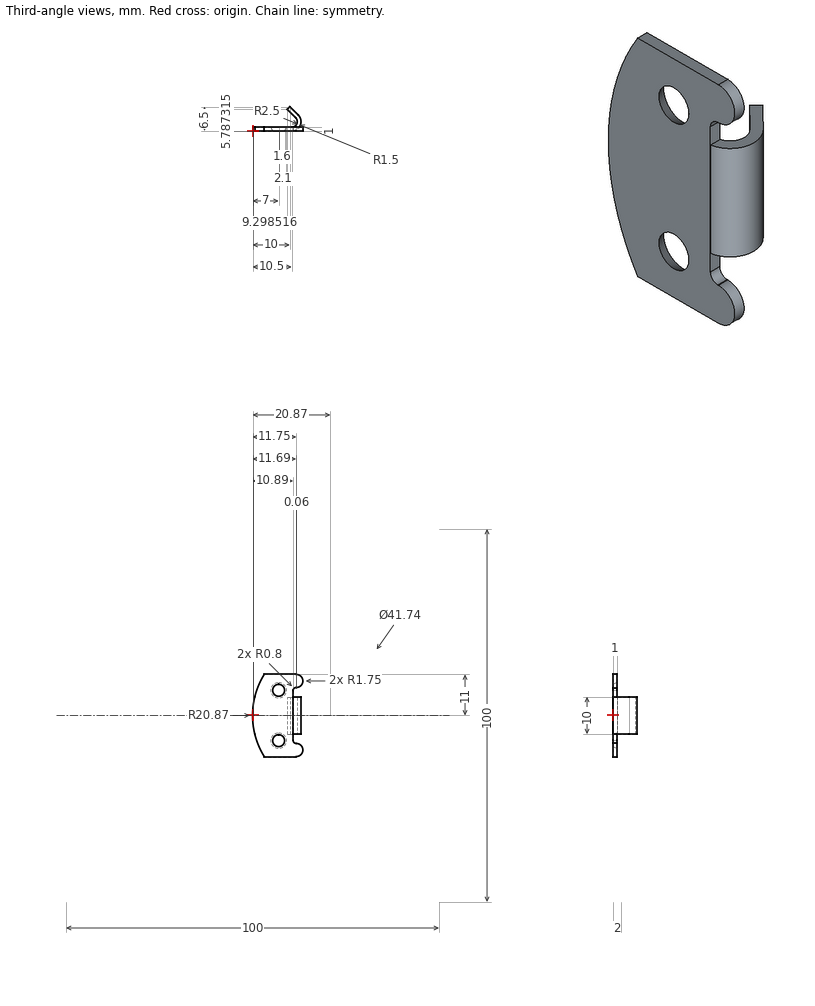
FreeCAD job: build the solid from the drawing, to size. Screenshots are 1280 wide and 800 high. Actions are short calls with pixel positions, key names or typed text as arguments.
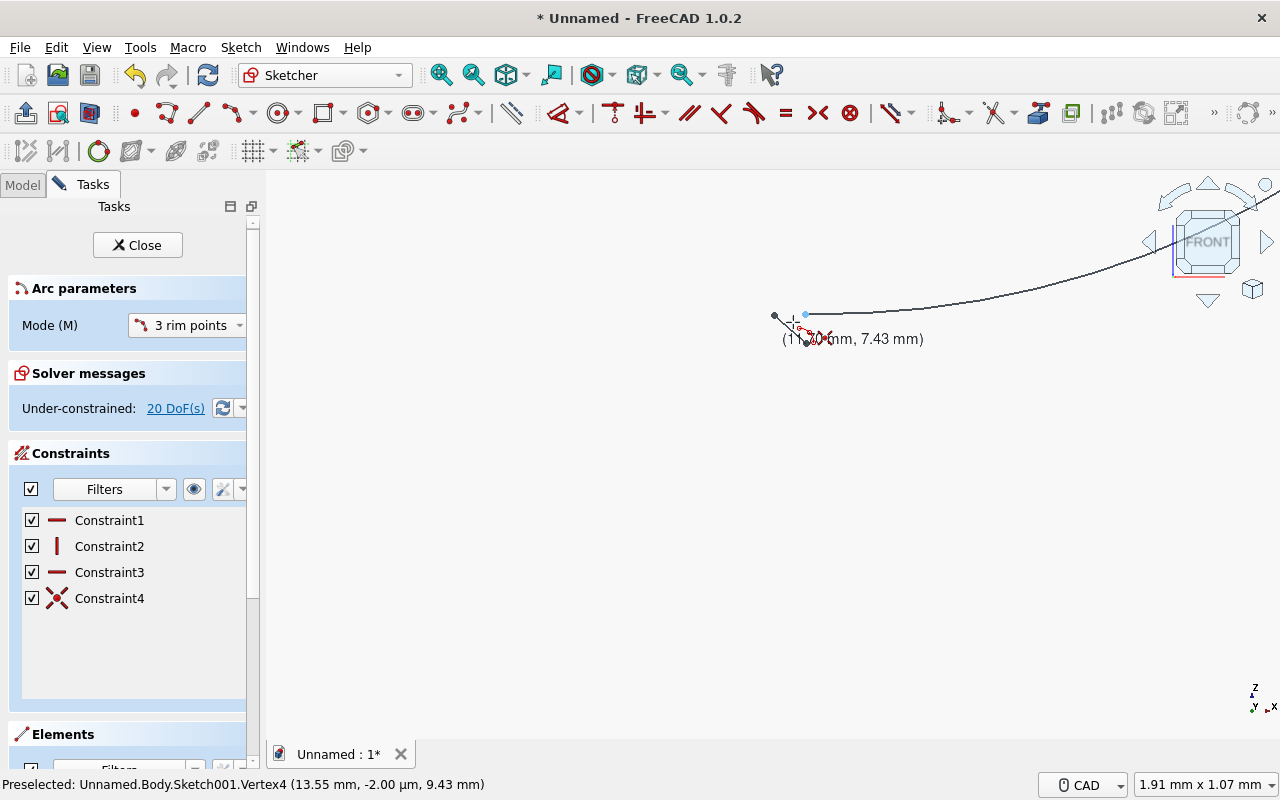
click(774, 315)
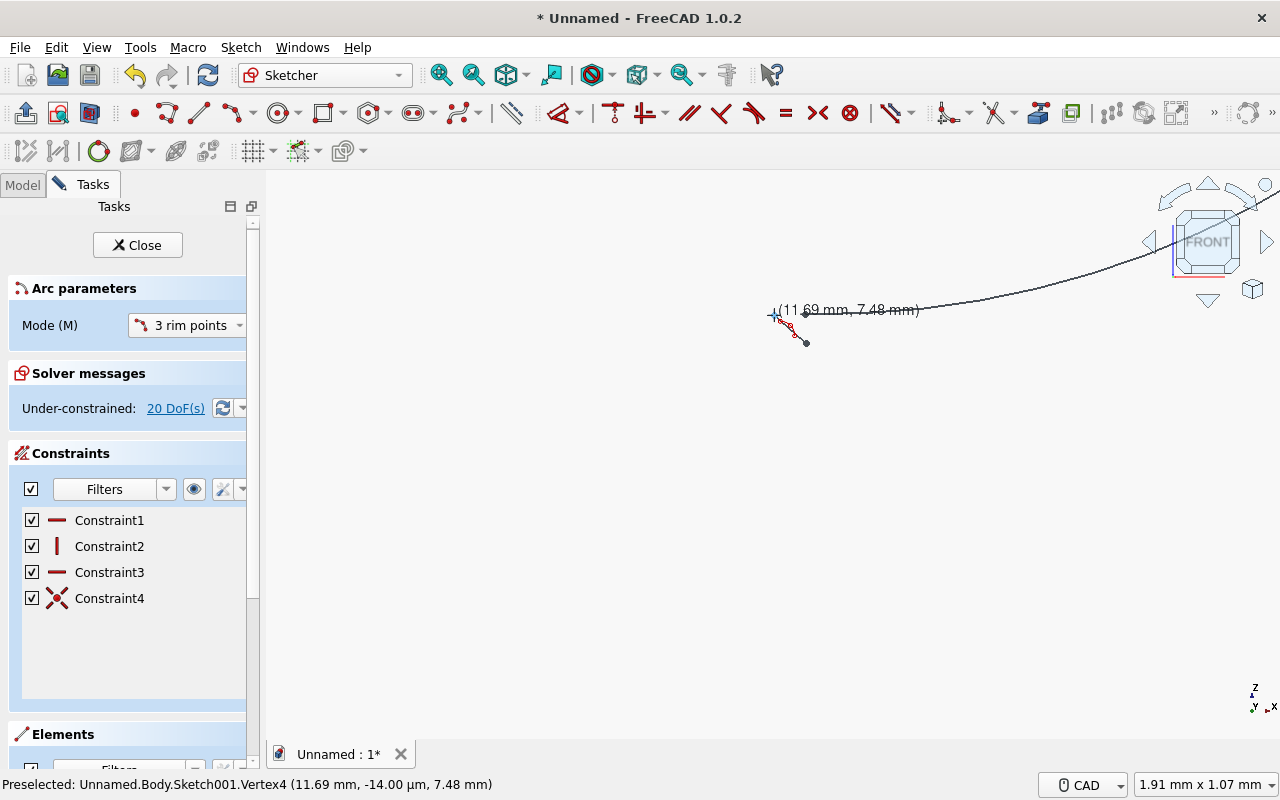
scroll(793, 322, down, 17)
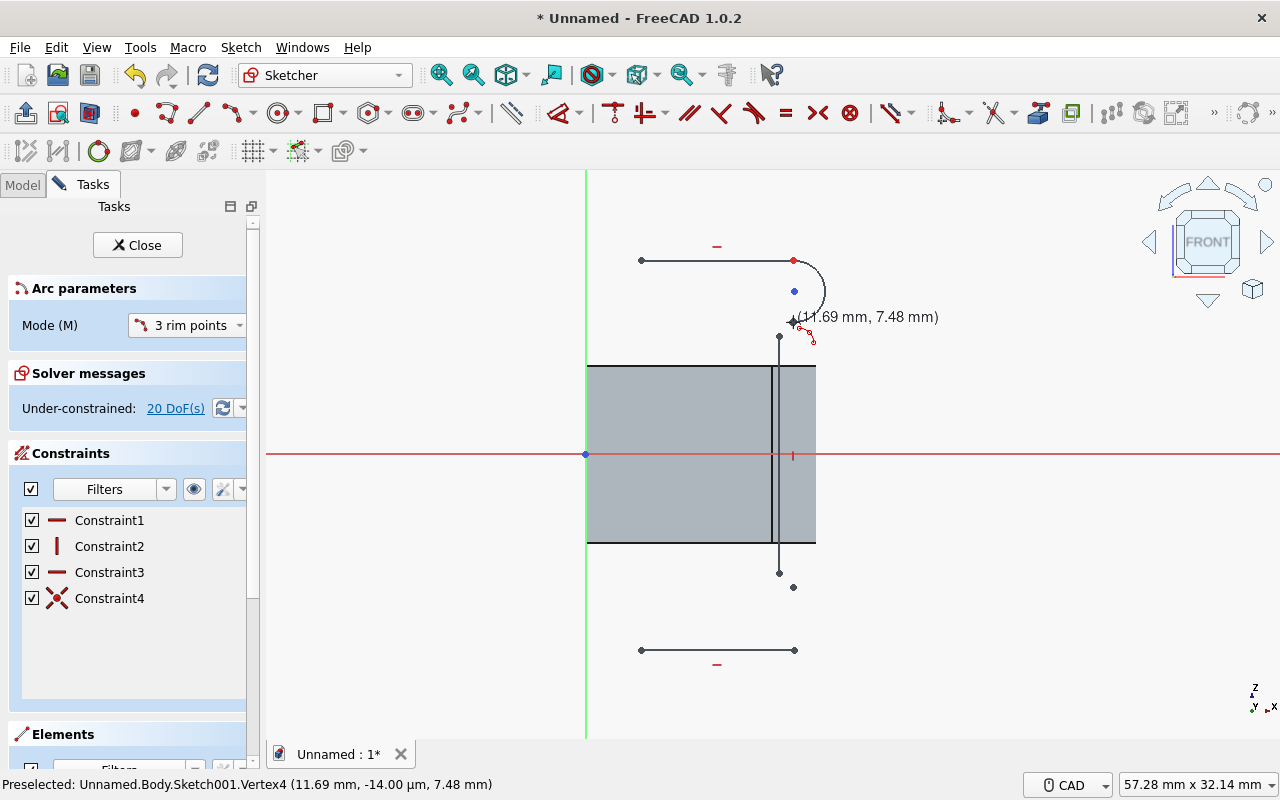
click(779, 337)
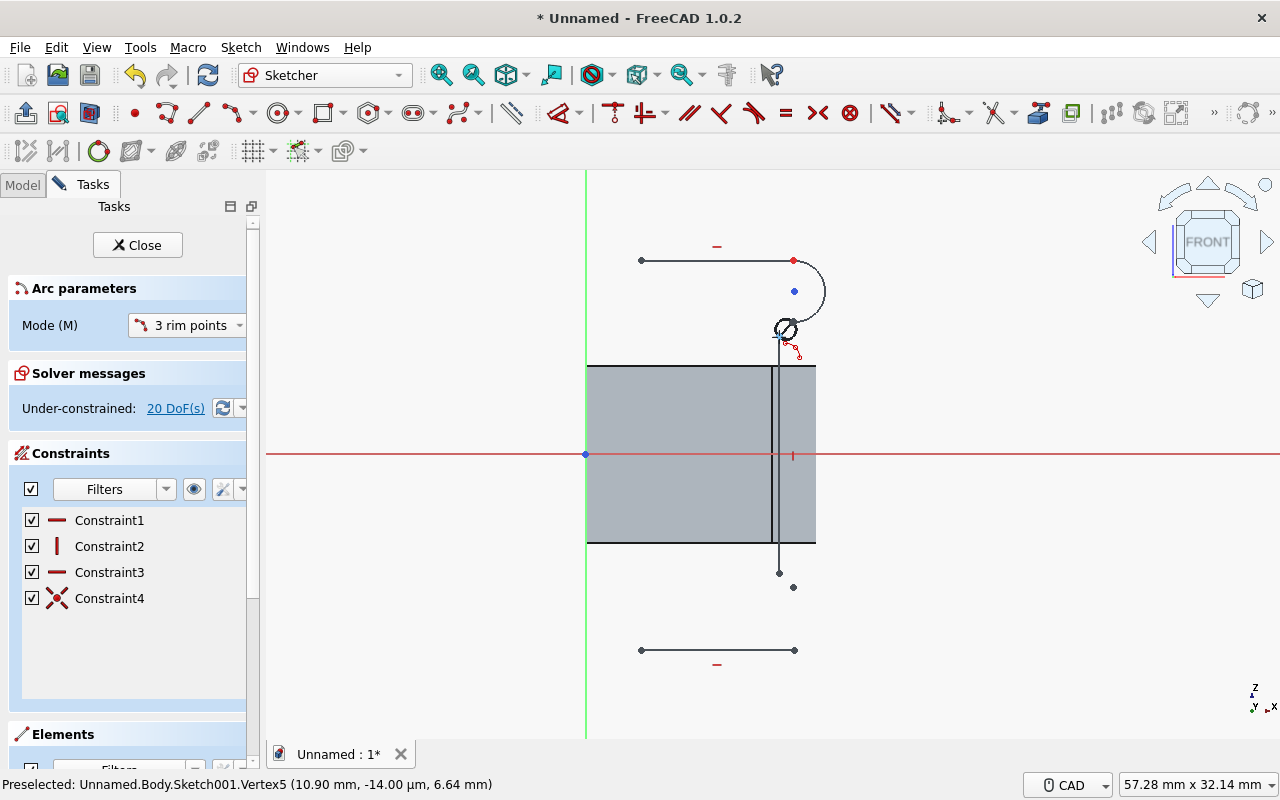
scroll(783, 326, up, 7)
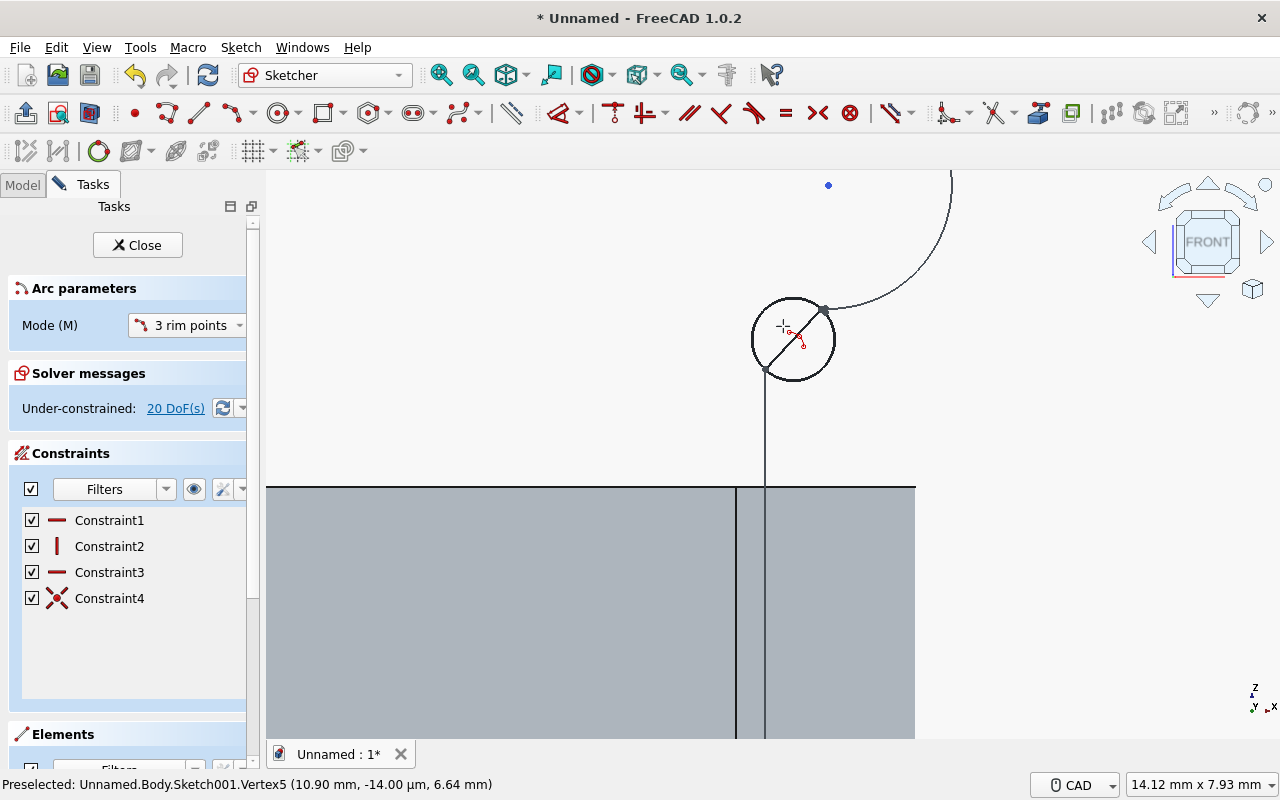
click(781, 325)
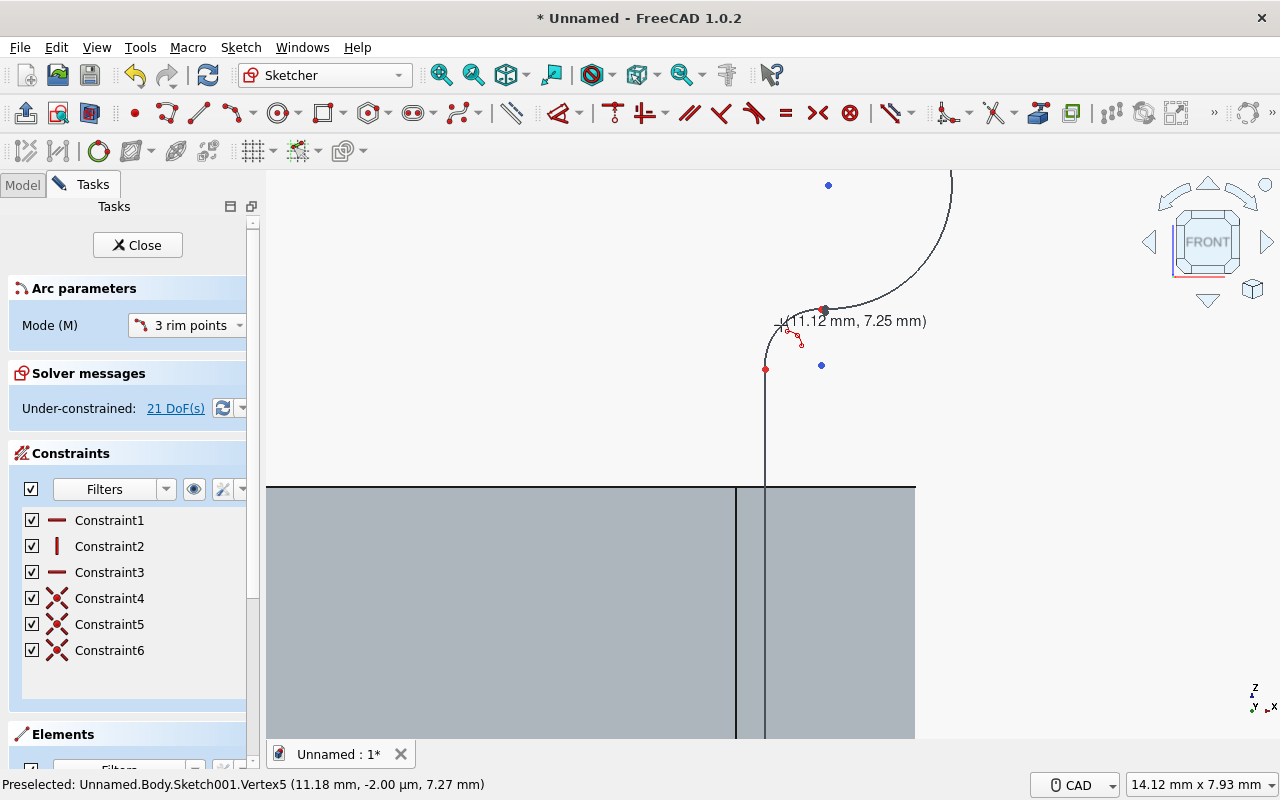
scroll(782, 326, down, 7)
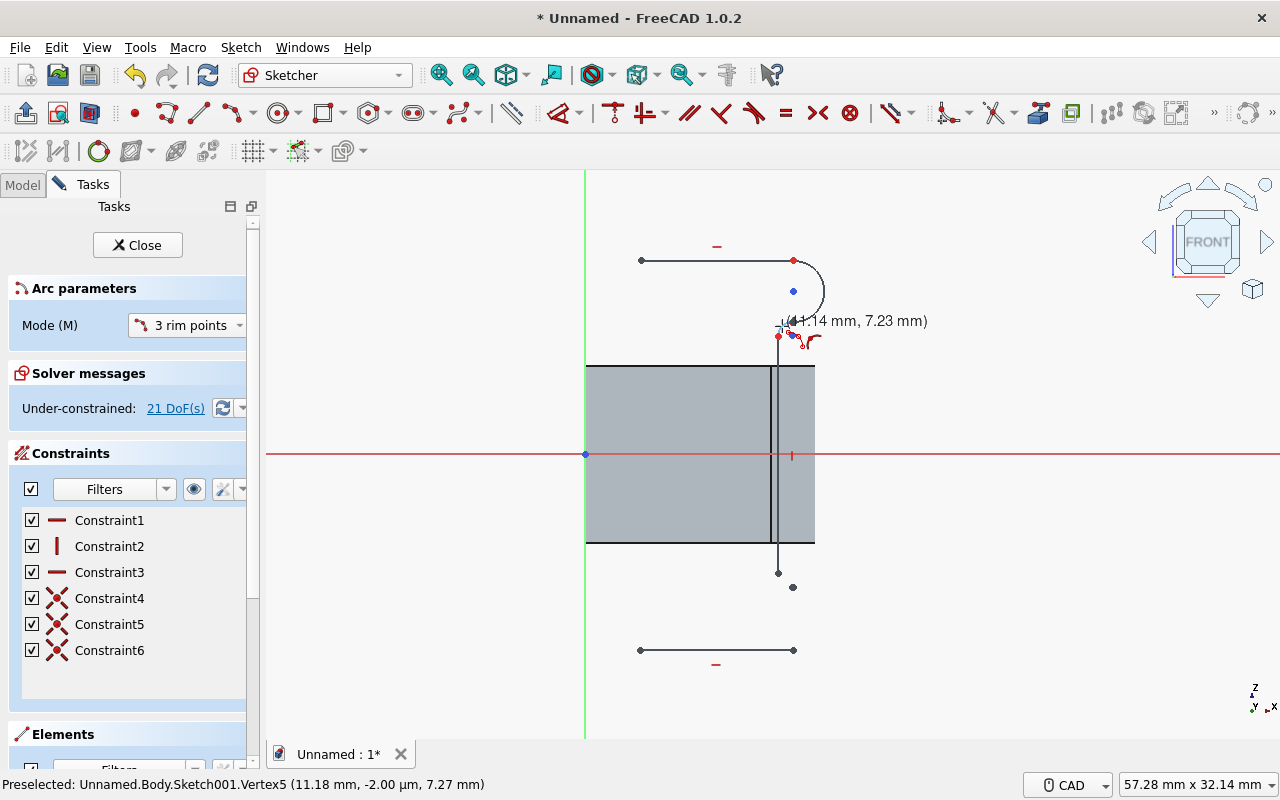
click(778, 574)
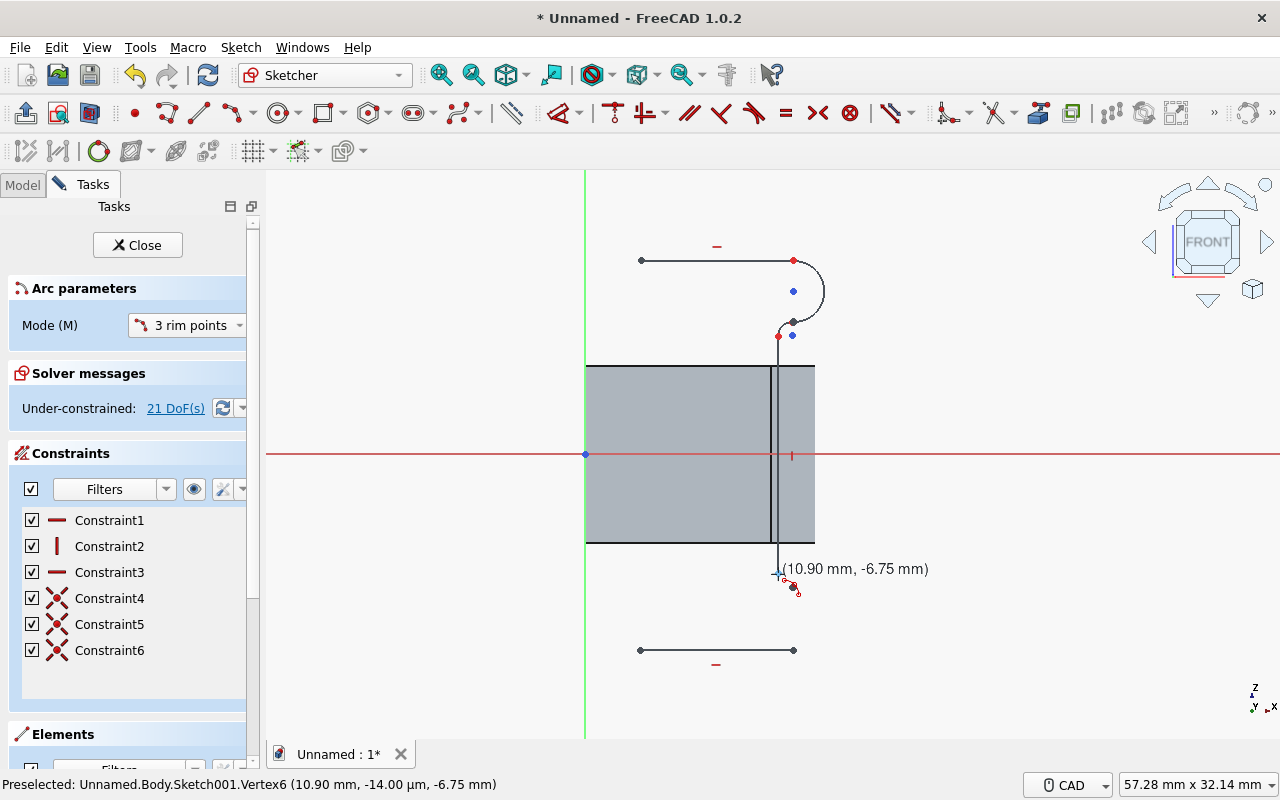
scroll(792, 587, up, 17)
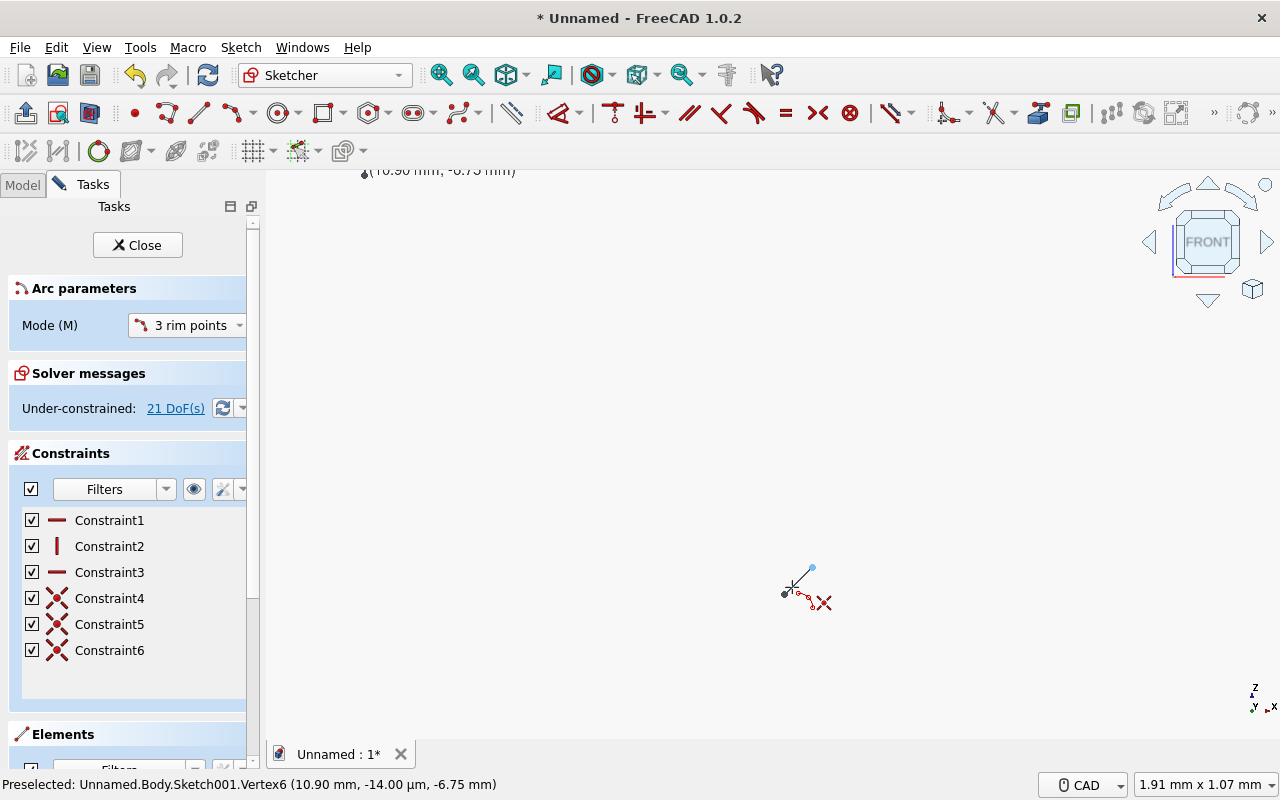
click(784, 565)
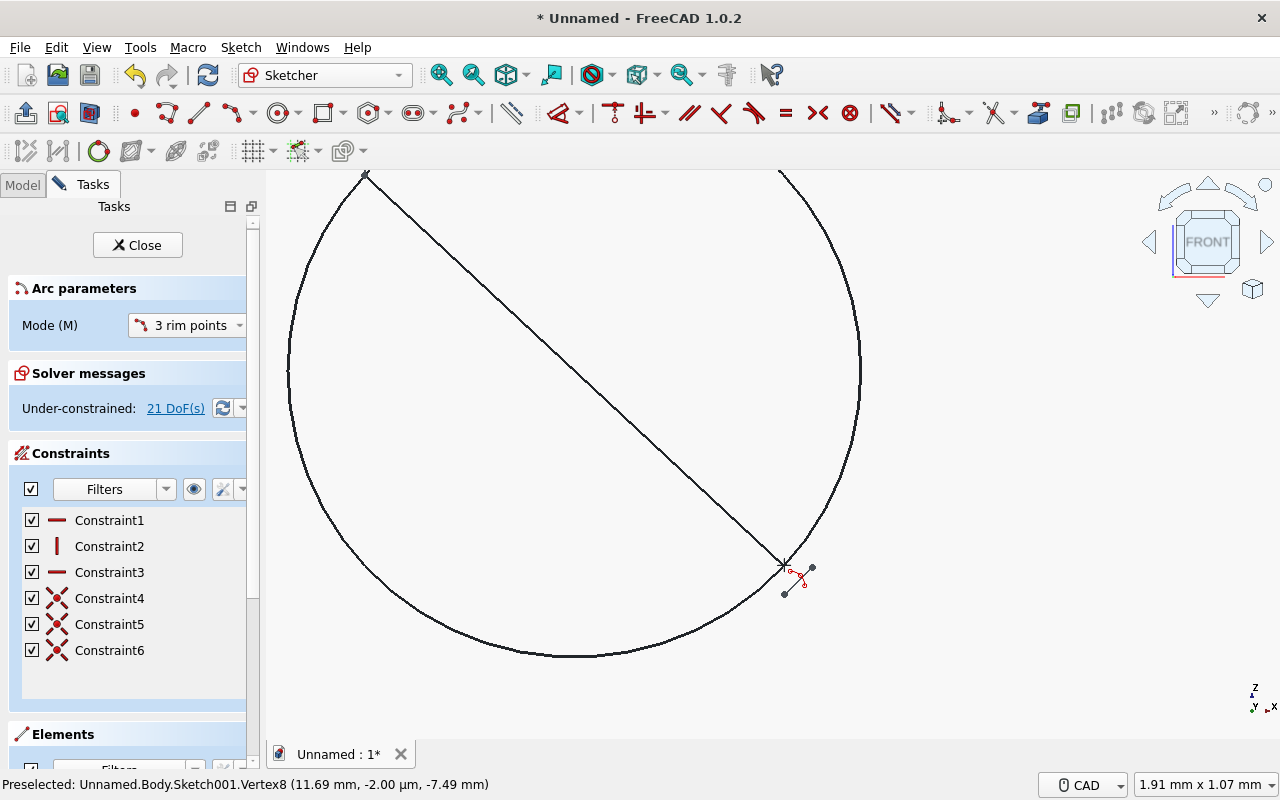
scroll(792, 588, down, 17)